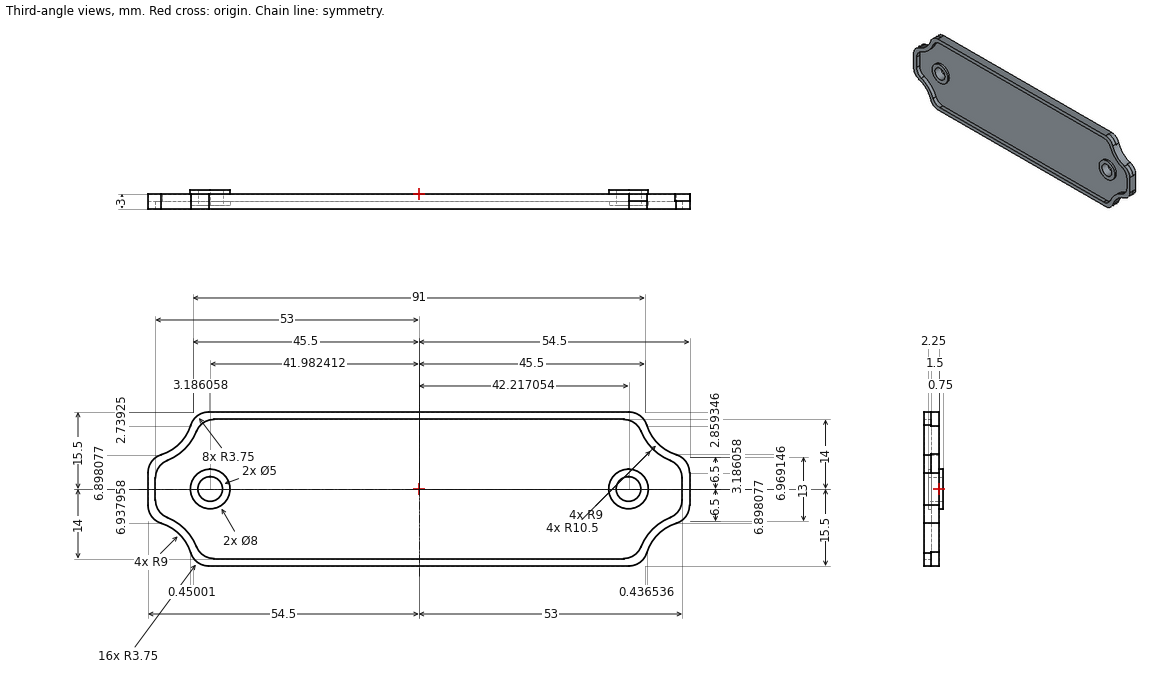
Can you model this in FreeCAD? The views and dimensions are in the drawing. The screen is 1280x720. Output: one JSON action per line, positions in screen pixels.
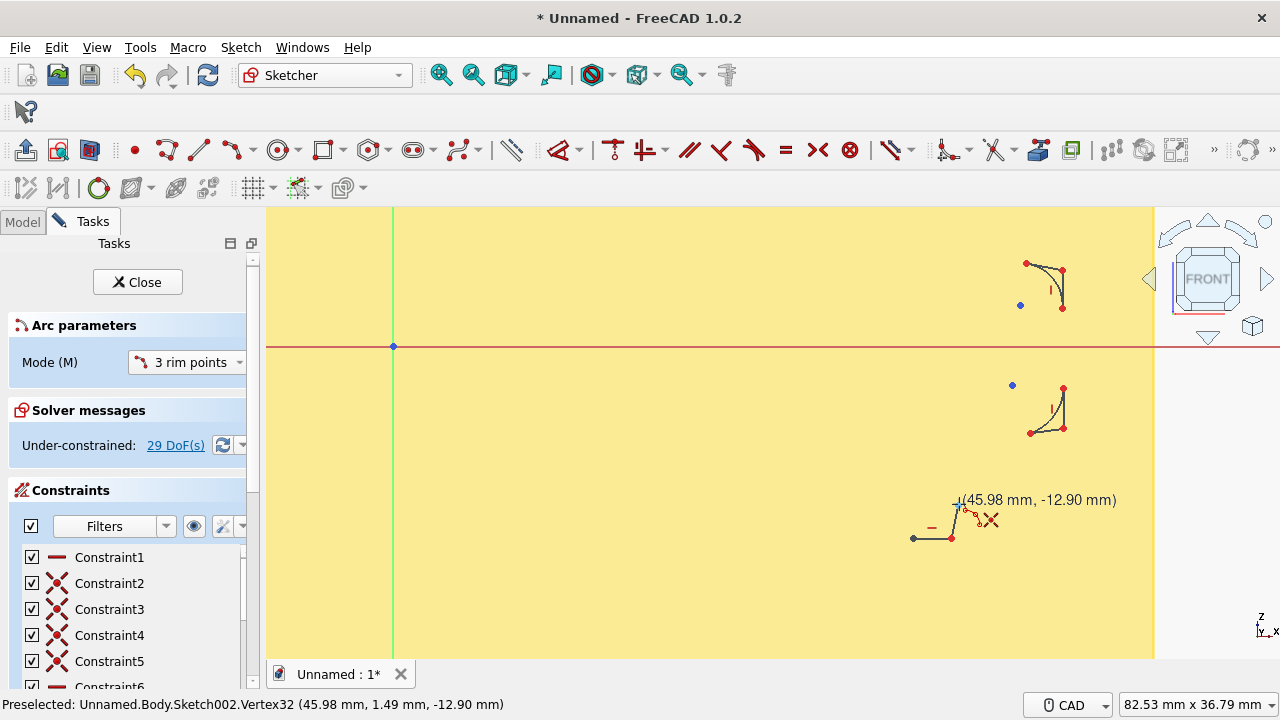
{"action": "left_click", "coordinate": [958, 505]}
{"action": "left_click", "coordinate": [914, 539]}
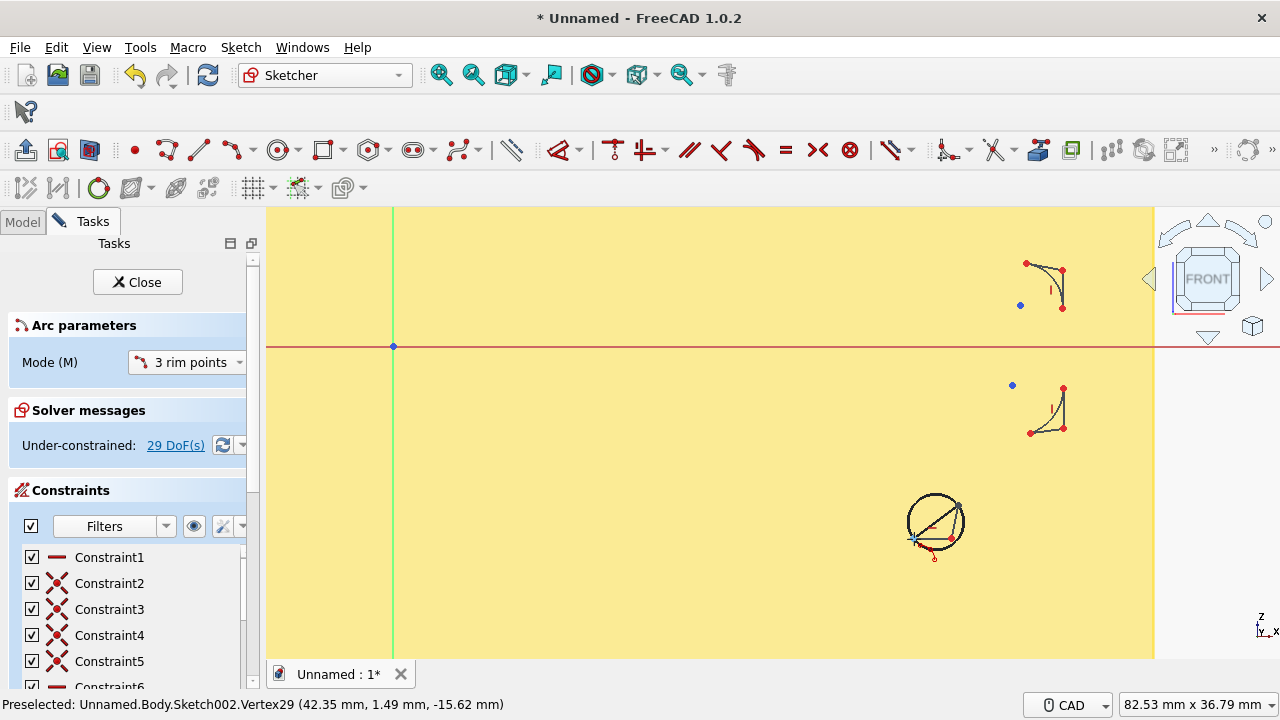
{"action": "scroll", "coordinate": [941, 528], "scroll_direction": "up", "scroll_amount": 3}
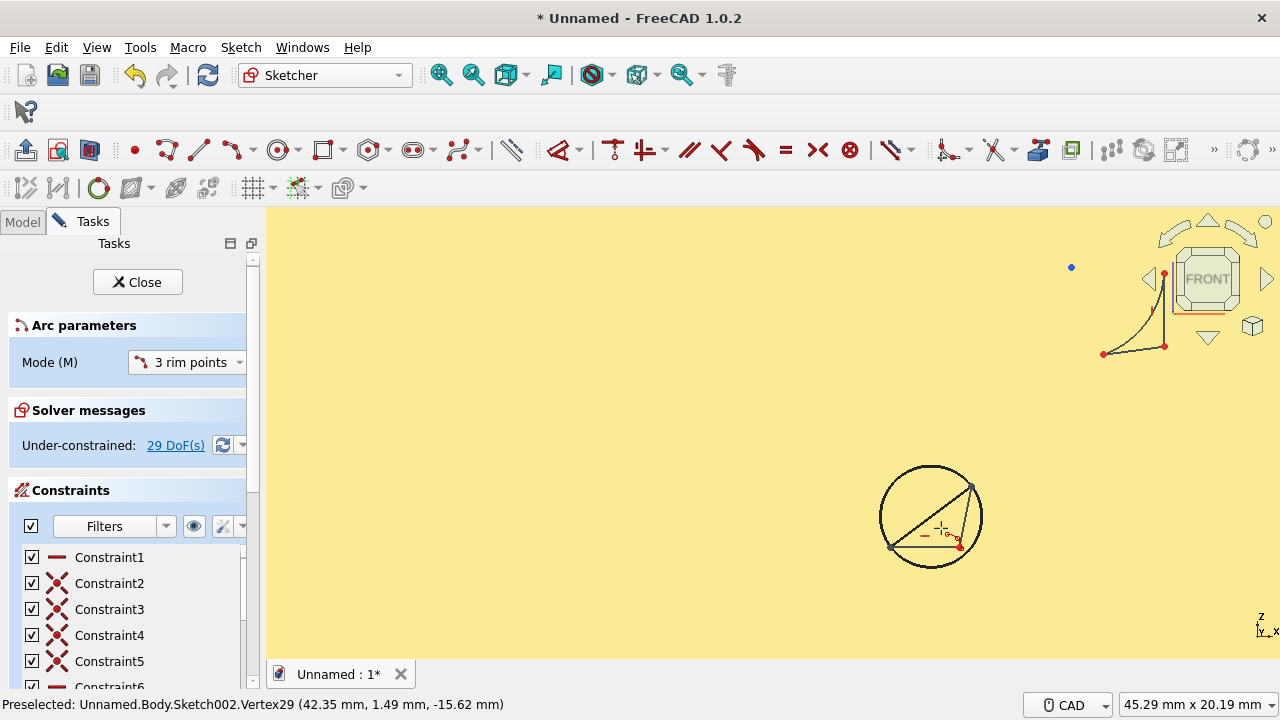
{"action": "left_click", "coordinate": [941, 527]}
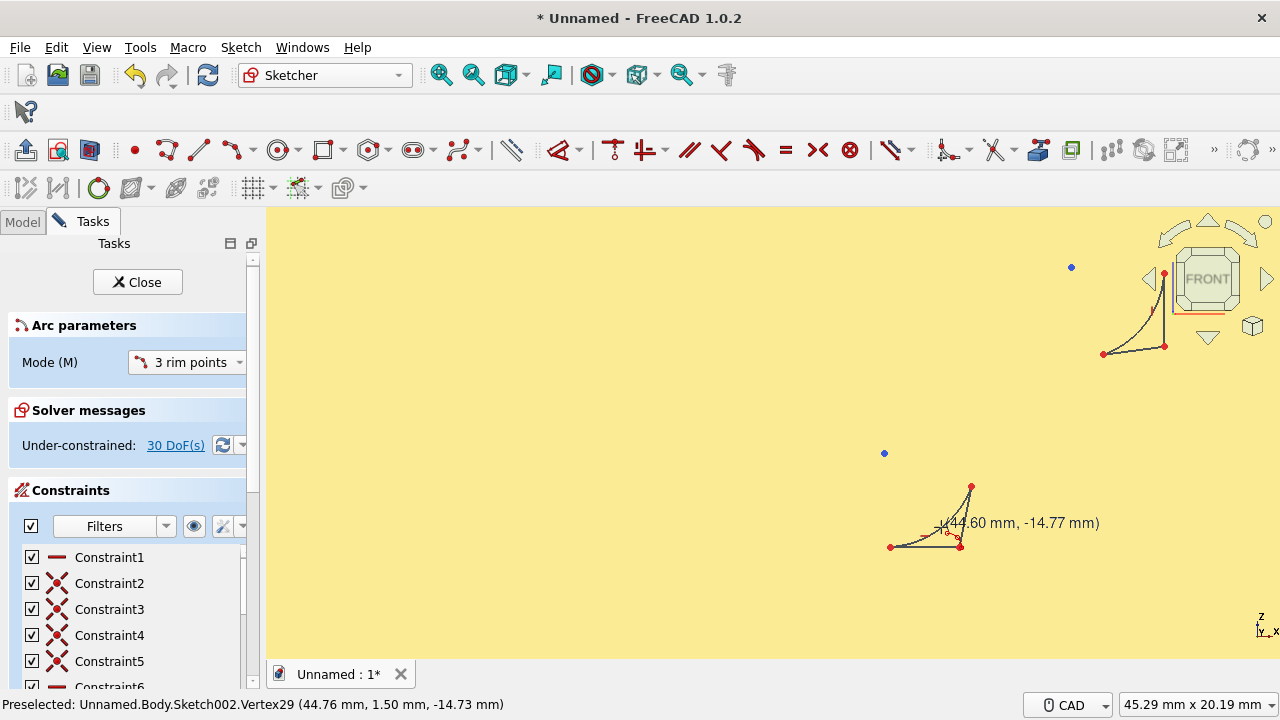
{"action": "left_click", "coordinate": [168, 150]}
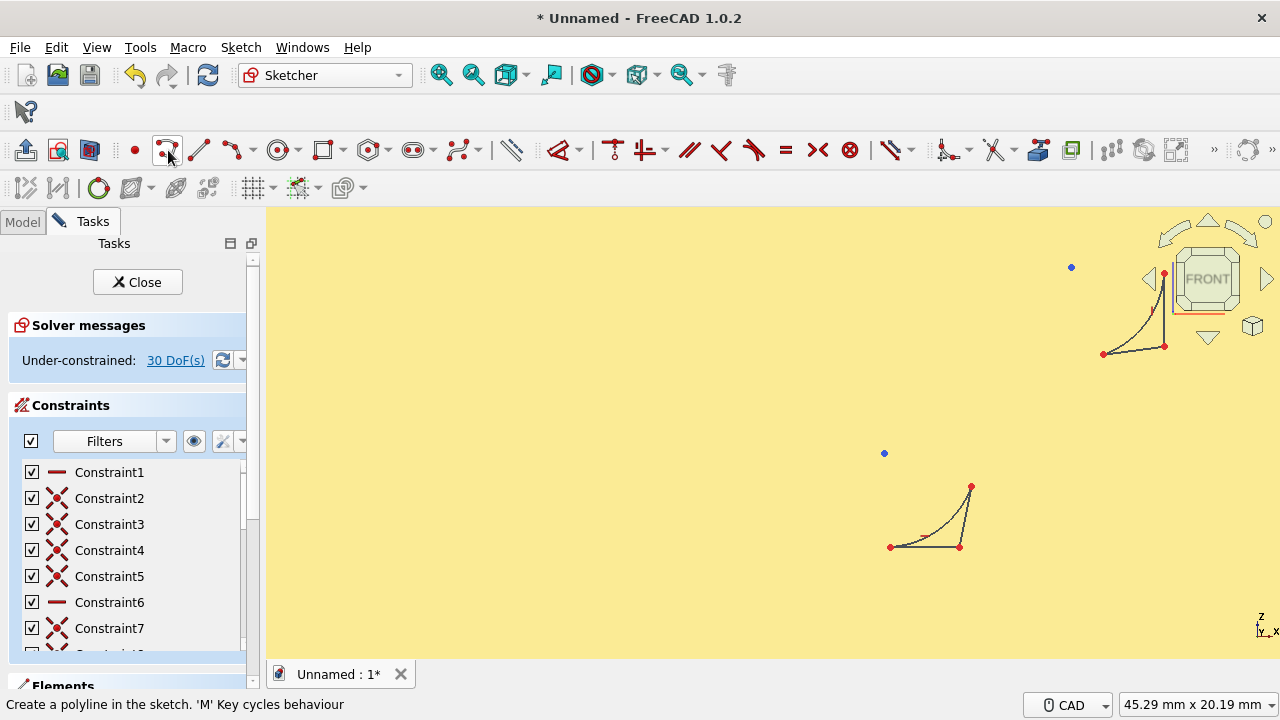
{"action": "scroll", "coordinate": [954, 510], "scroll_direction": "down", "scroll_amount": 7}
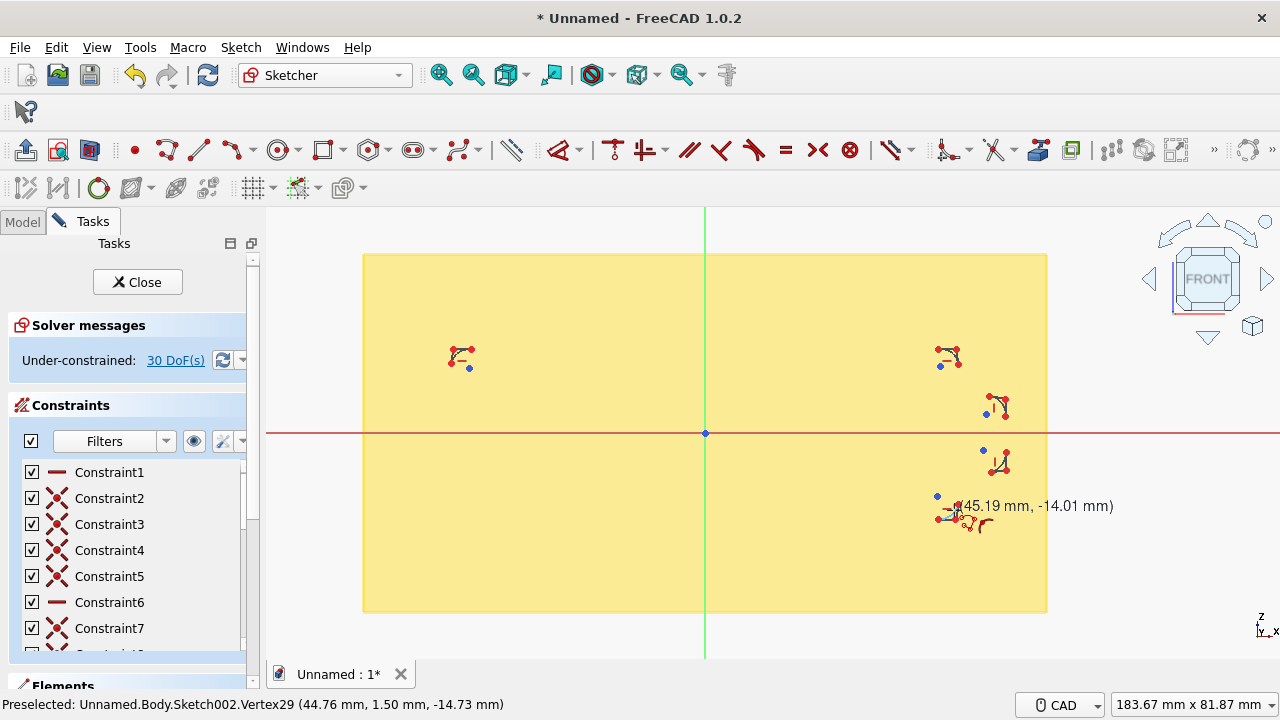
{"action": "left_click", "coordinate": [451, 503]}
{"action": "left_click", "coordinate": [454, 519]}
{"action": "left_click", "coordinate": [471, 519]}
{"action": "right_click", "coordinate": [471, 519]}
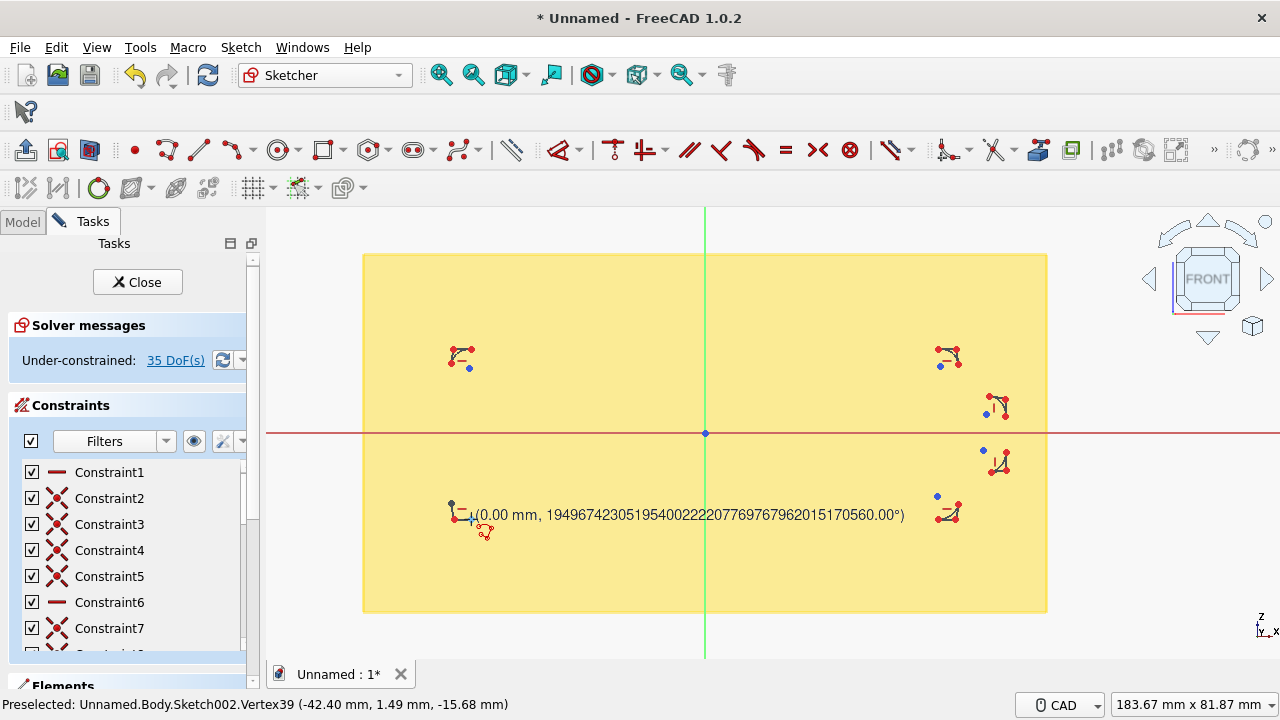
{"action": "left_click", "coordinate": [232, 150]}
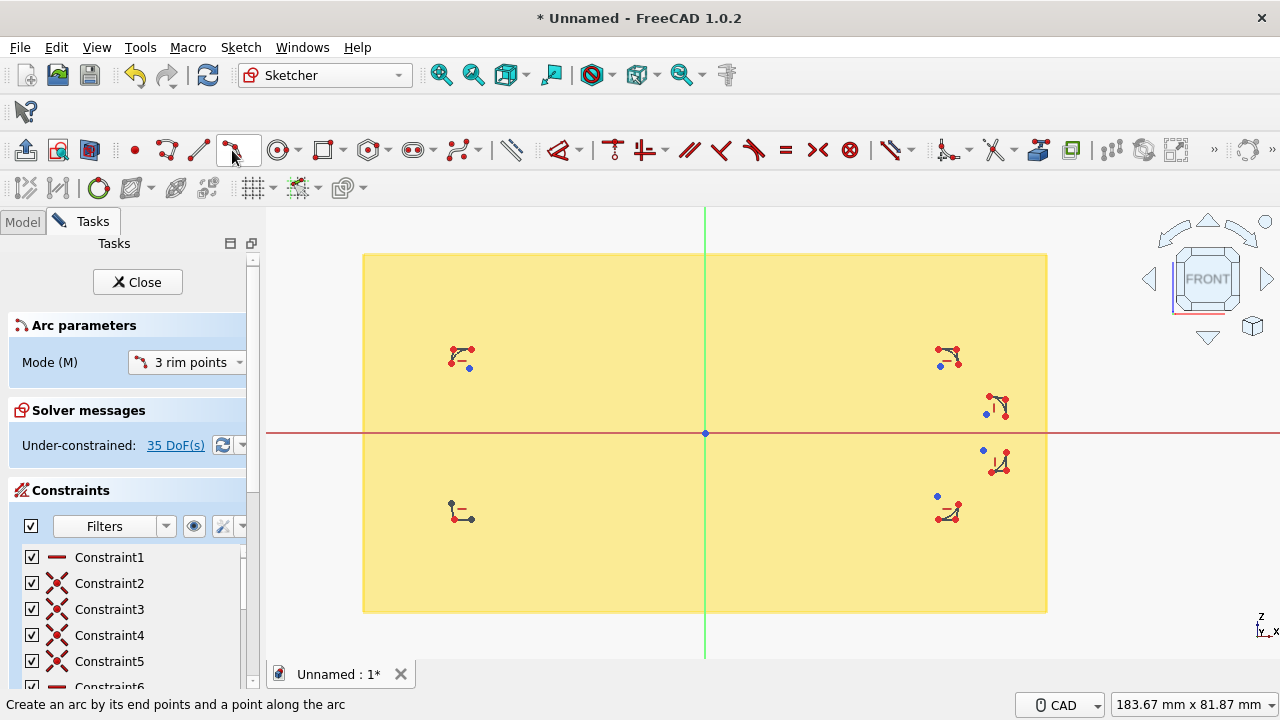
{"action": "scroll", "coordinate": [471, 519], "scroll_direction": "up", "scroll_amount": 3}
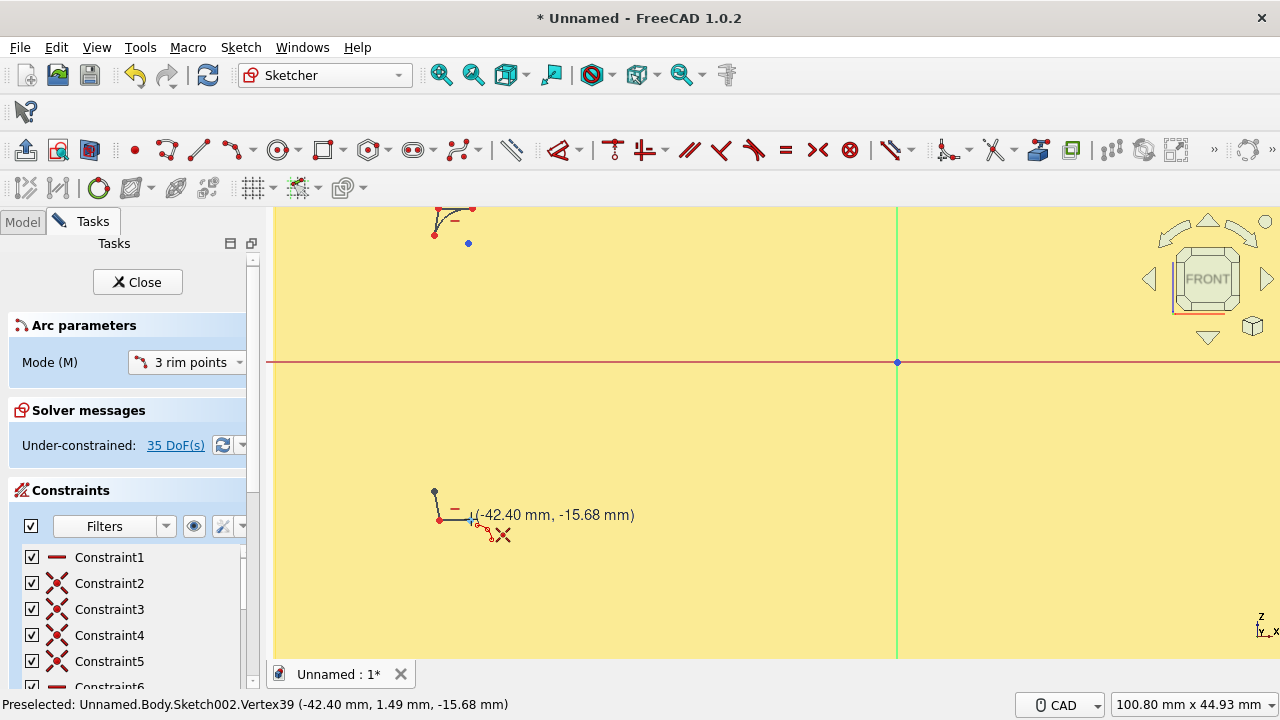
{"action": "left_click", "coordinate": [471, 520]}
{"action": "left_click", "coordinate": [434, 491]}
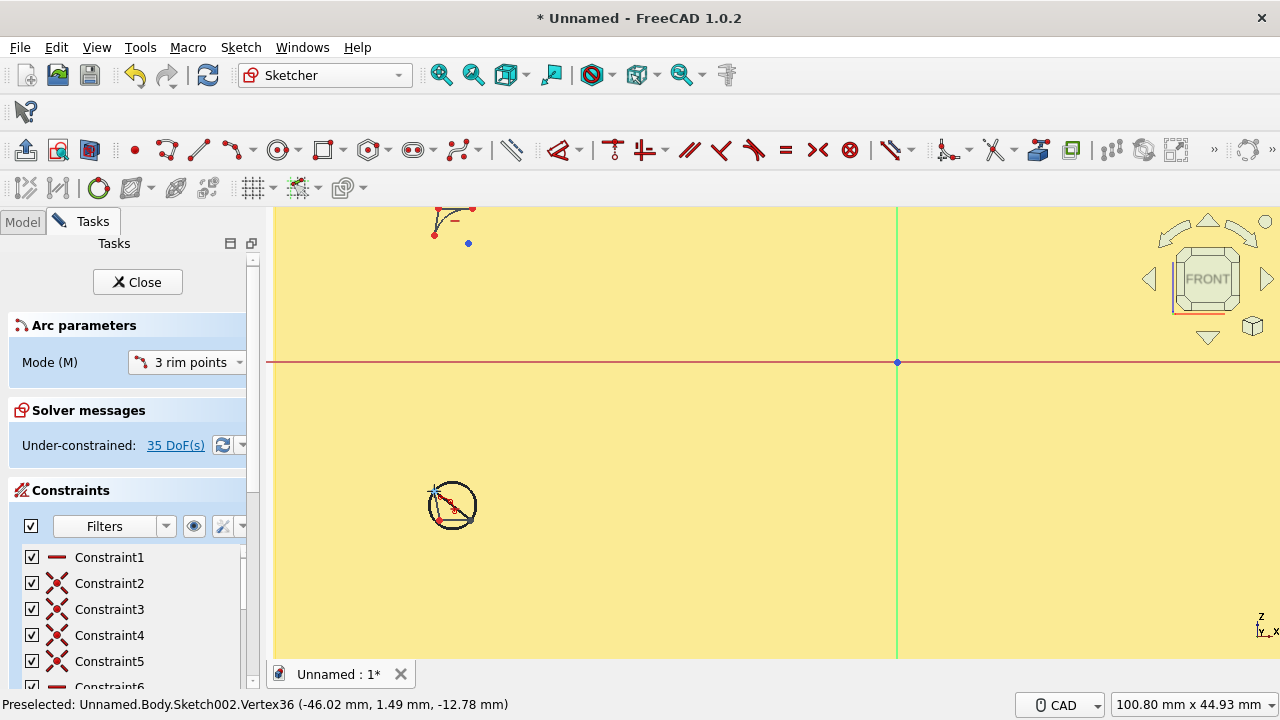
{"action": "scroll", "coordinate": [448, 510], "scroll_direction": "up", "scroll_amount": 4}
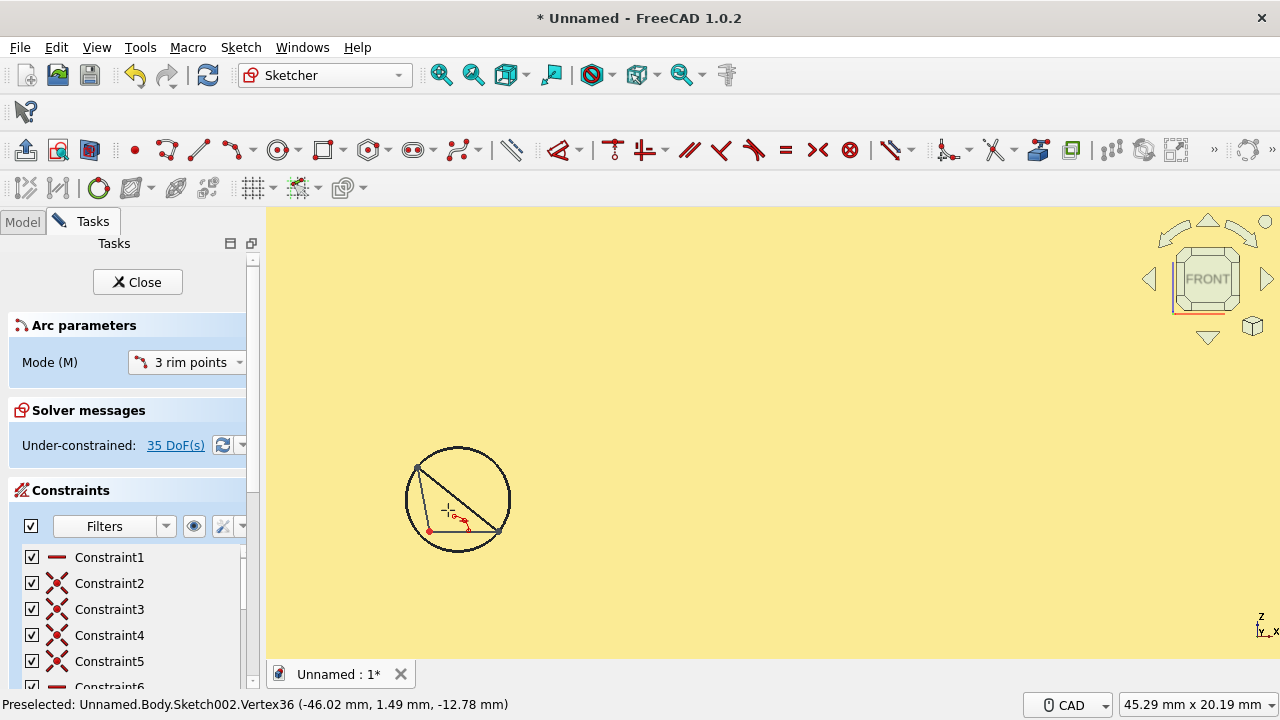
{"action": "left_click", "coordinate": [449, 510]}